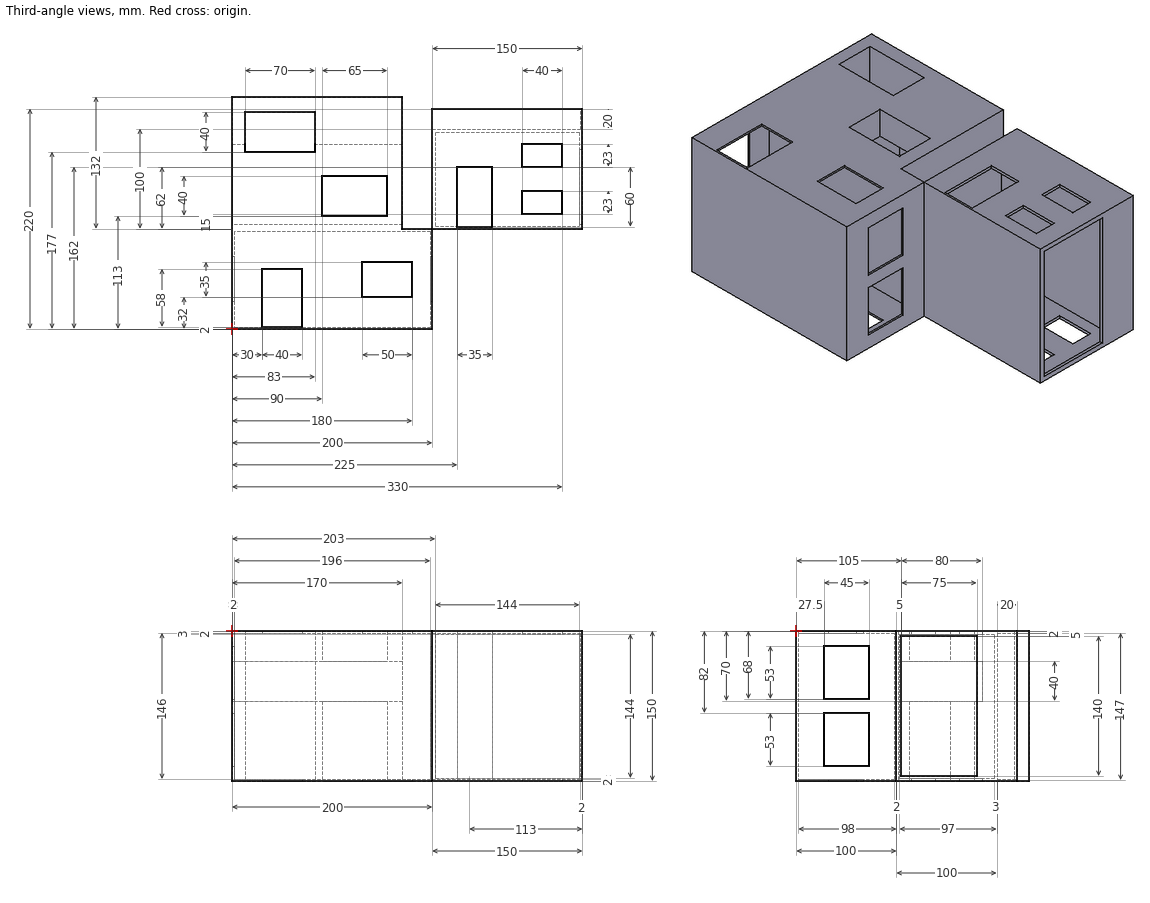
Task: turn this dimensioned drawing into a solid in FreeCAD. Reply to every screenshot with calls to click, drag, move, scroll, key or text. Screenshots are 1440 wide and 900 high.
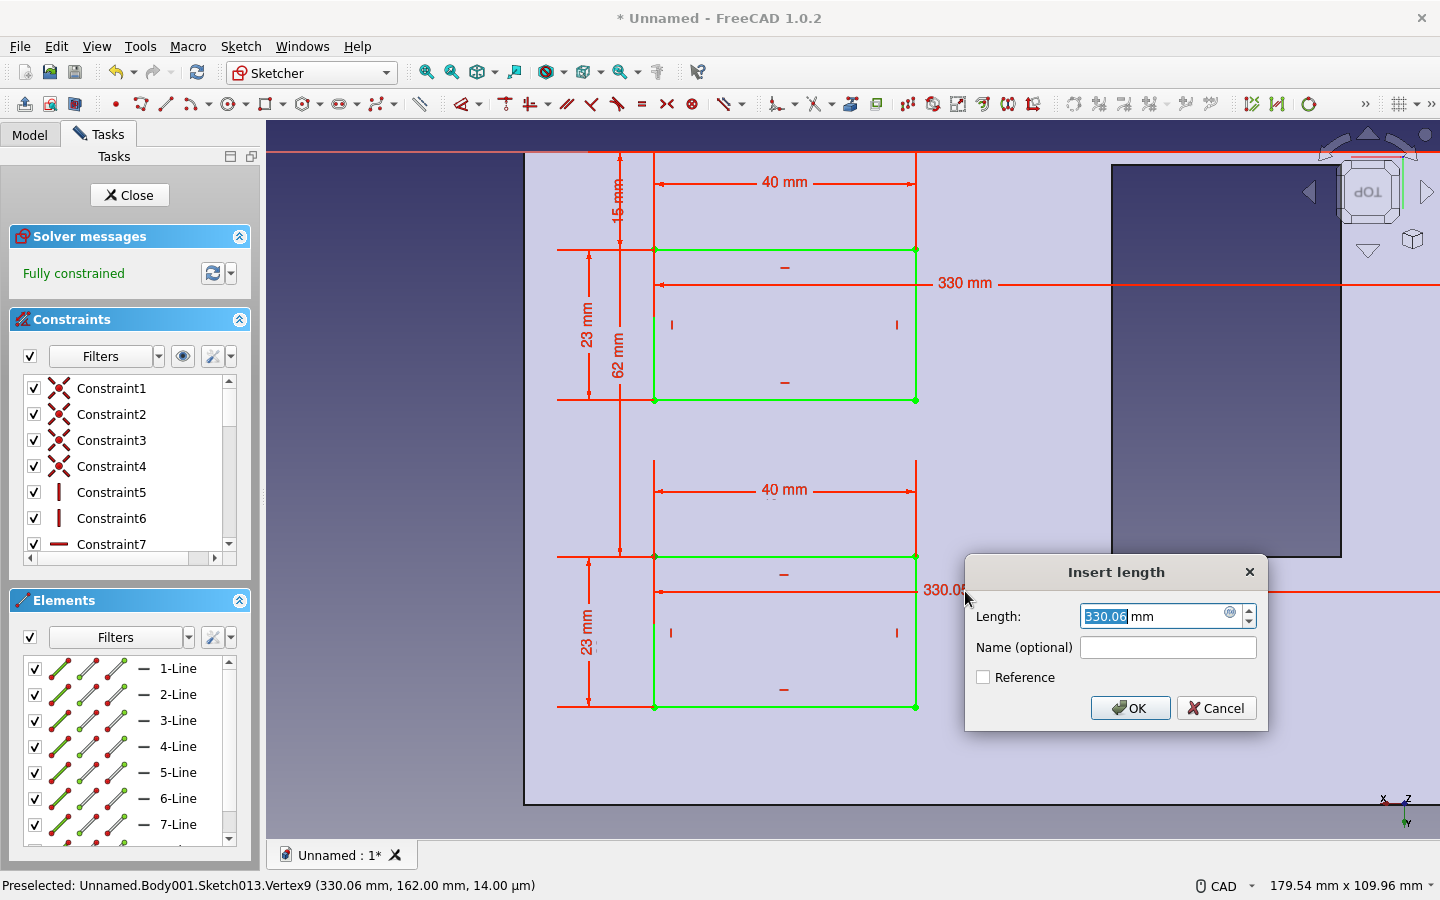
text(330)
key(Return)
key(Escape)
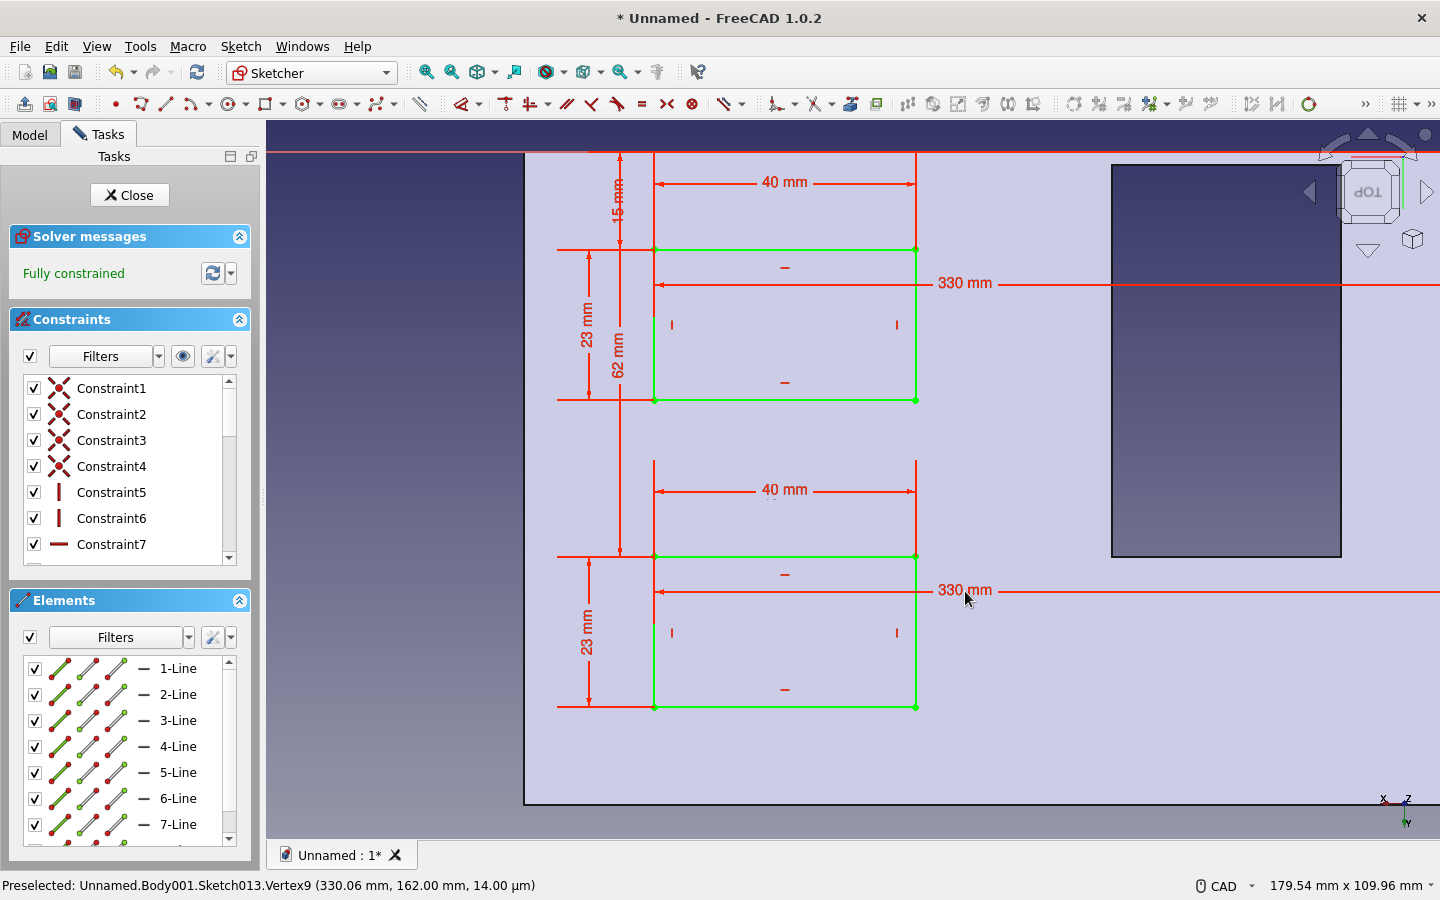
click(130, 195)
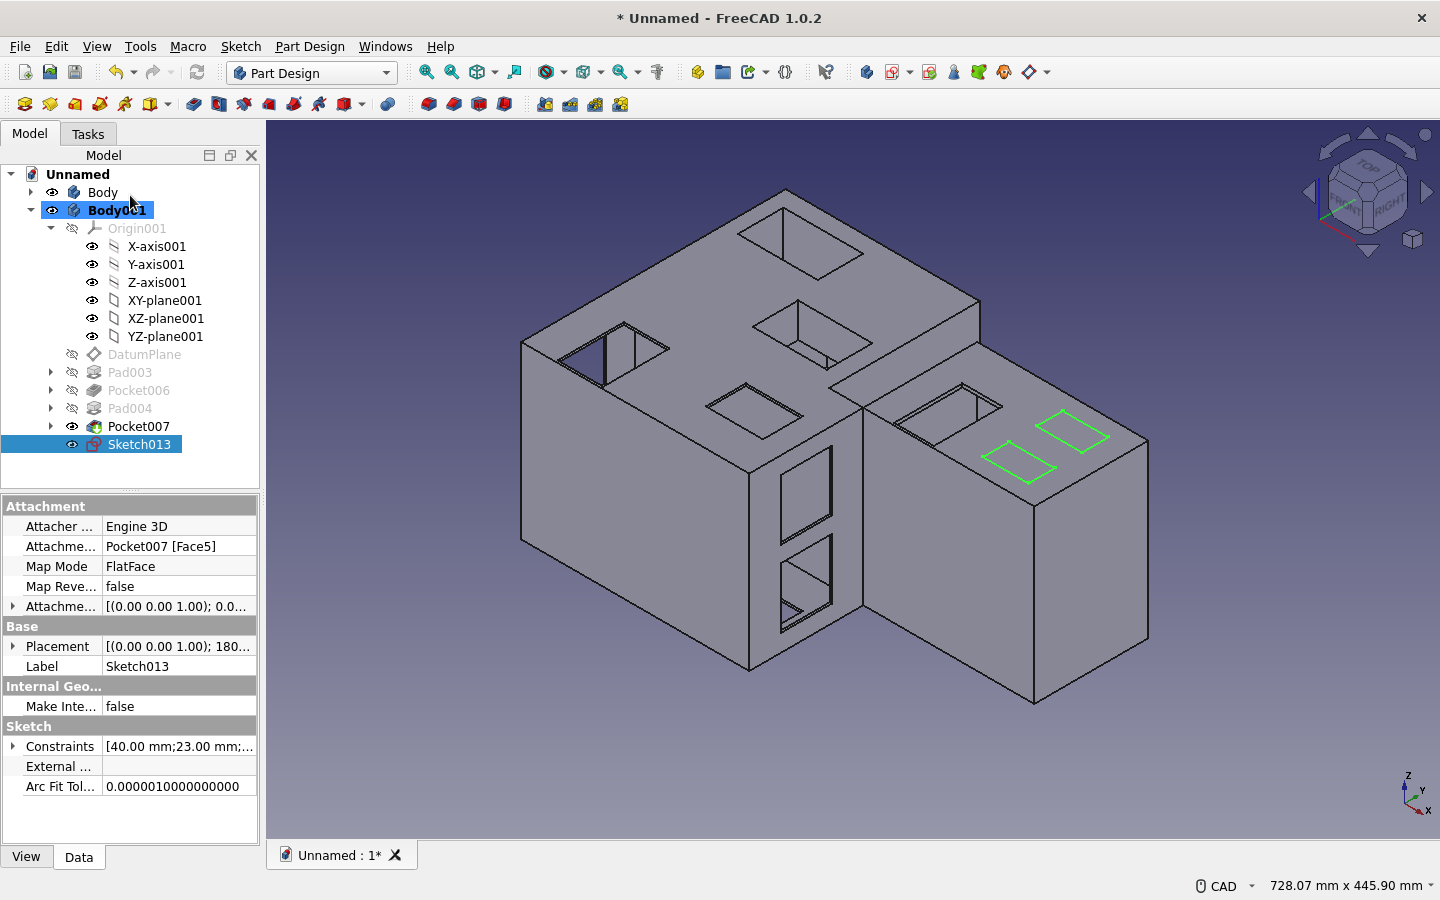
click(194, 104)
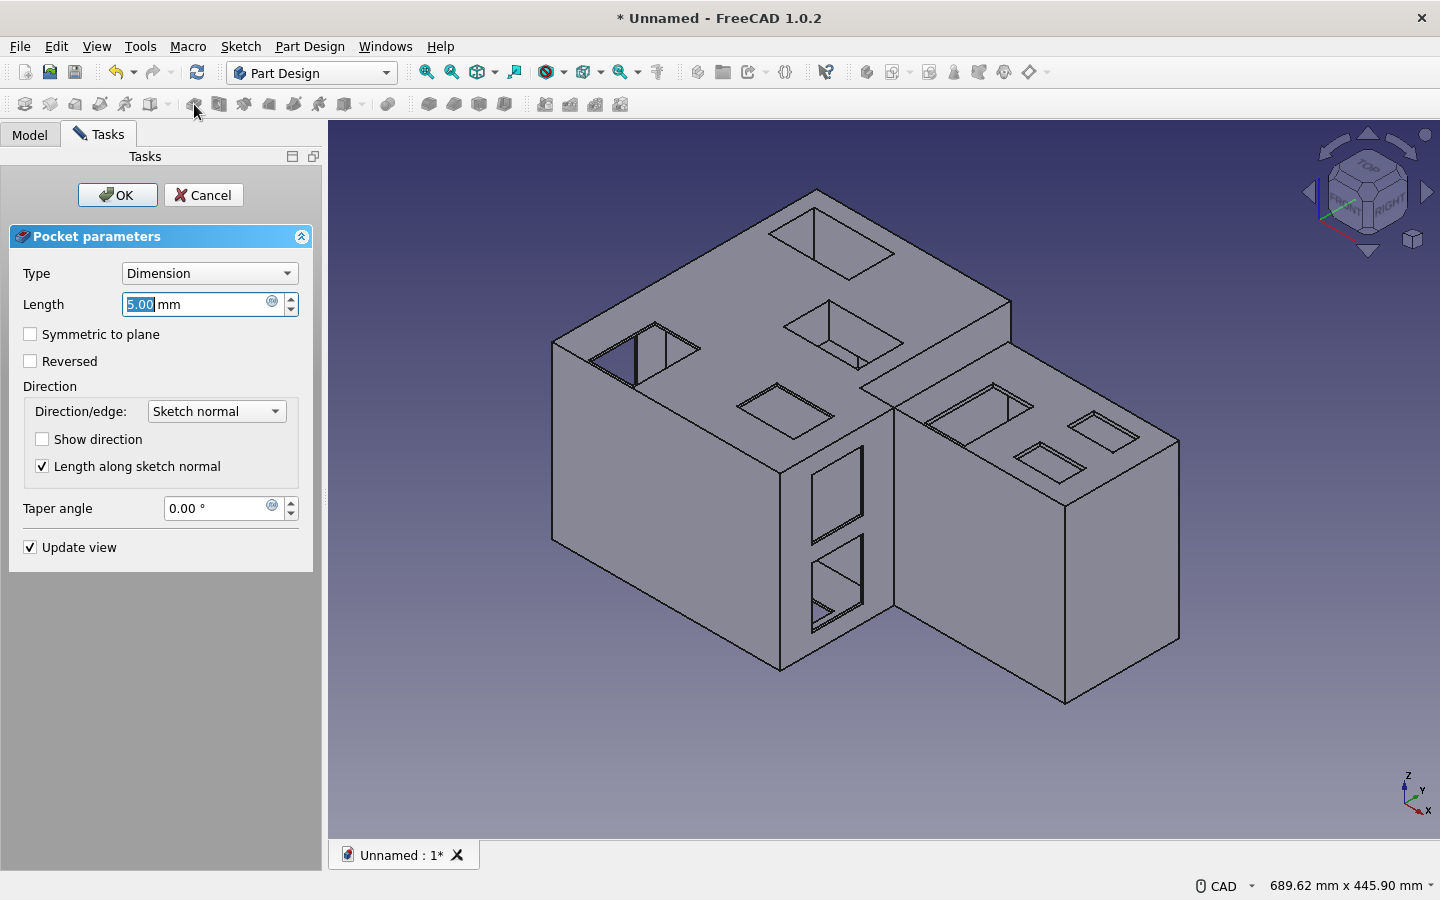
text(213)
key(Tab)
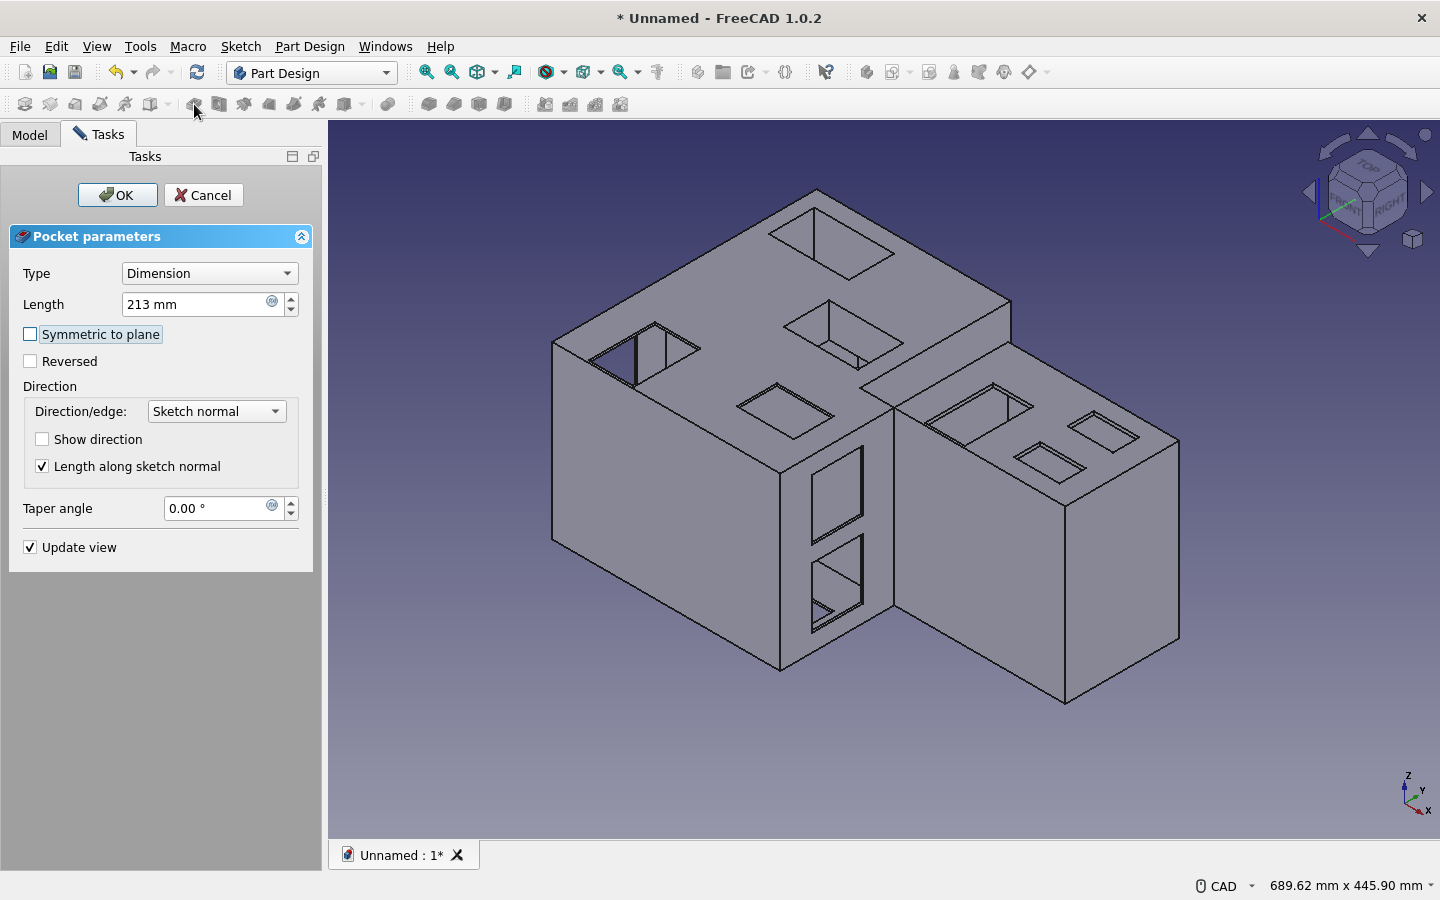
click(118, 195)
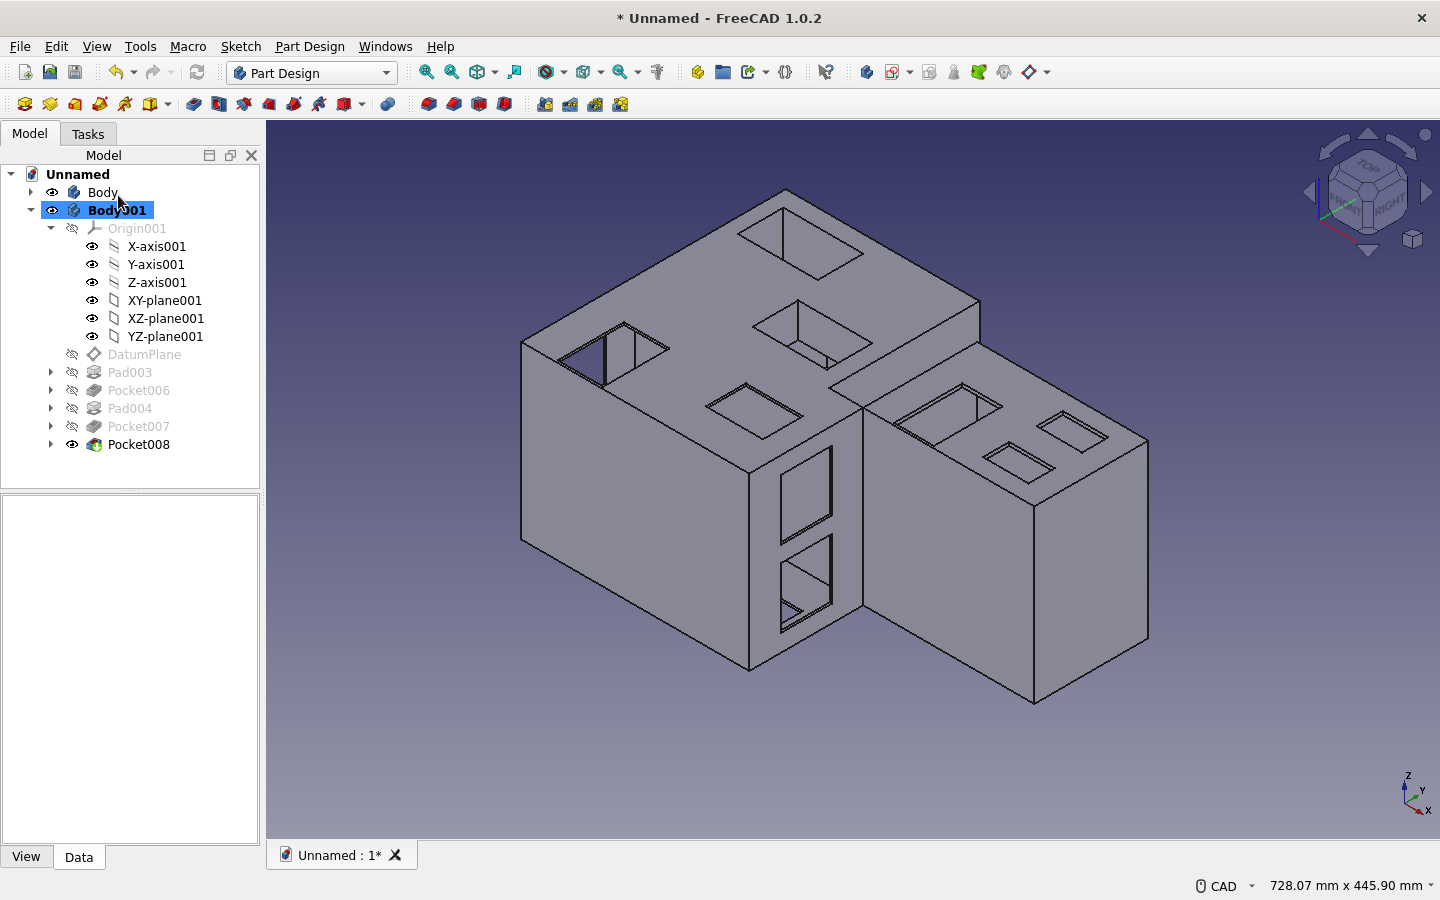
click(1091, 571)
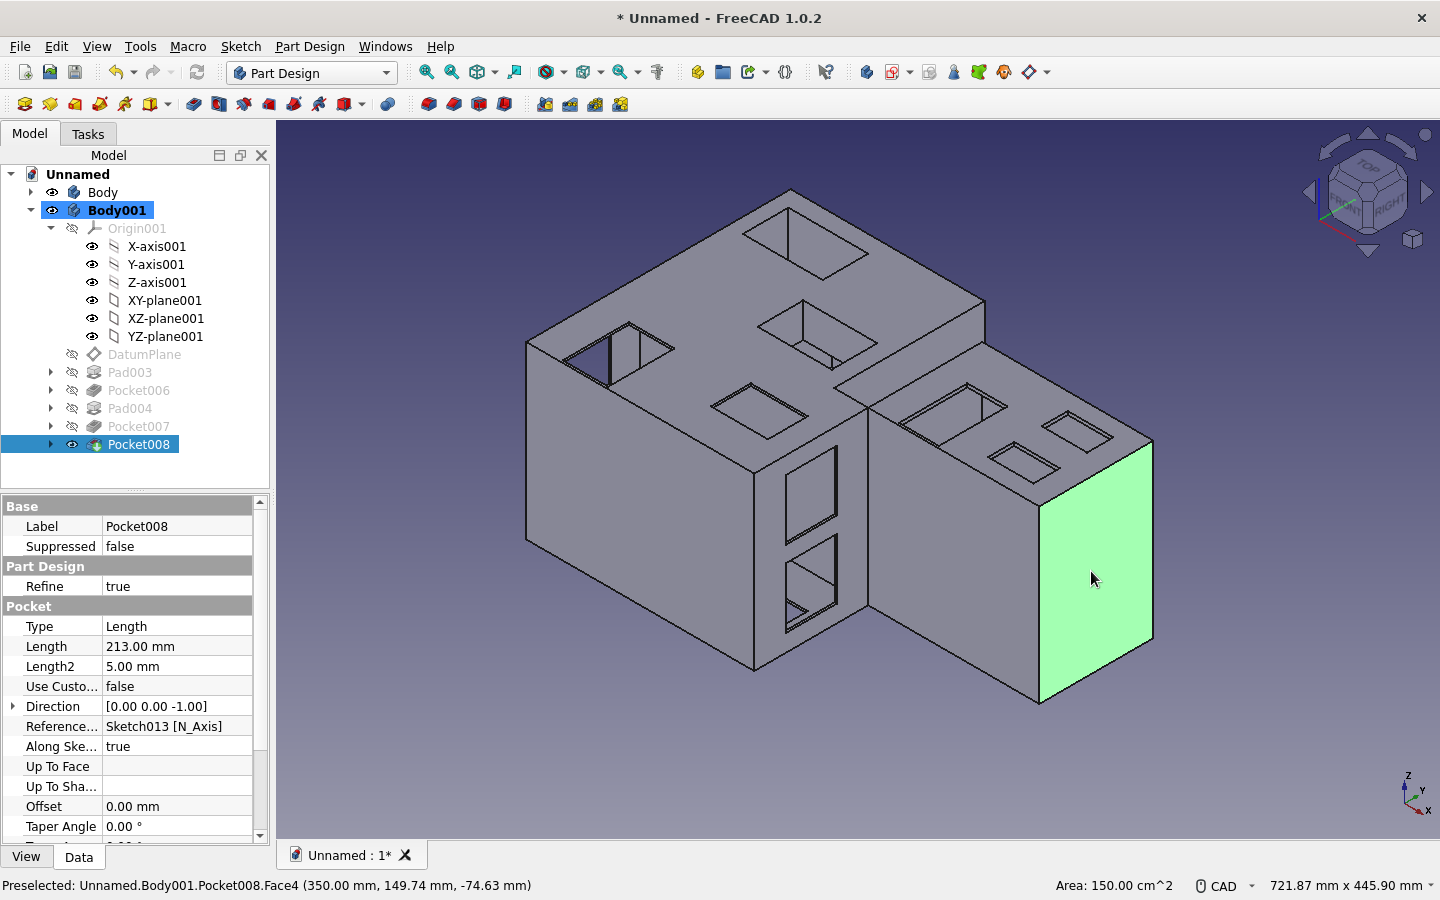
click(892, 72)